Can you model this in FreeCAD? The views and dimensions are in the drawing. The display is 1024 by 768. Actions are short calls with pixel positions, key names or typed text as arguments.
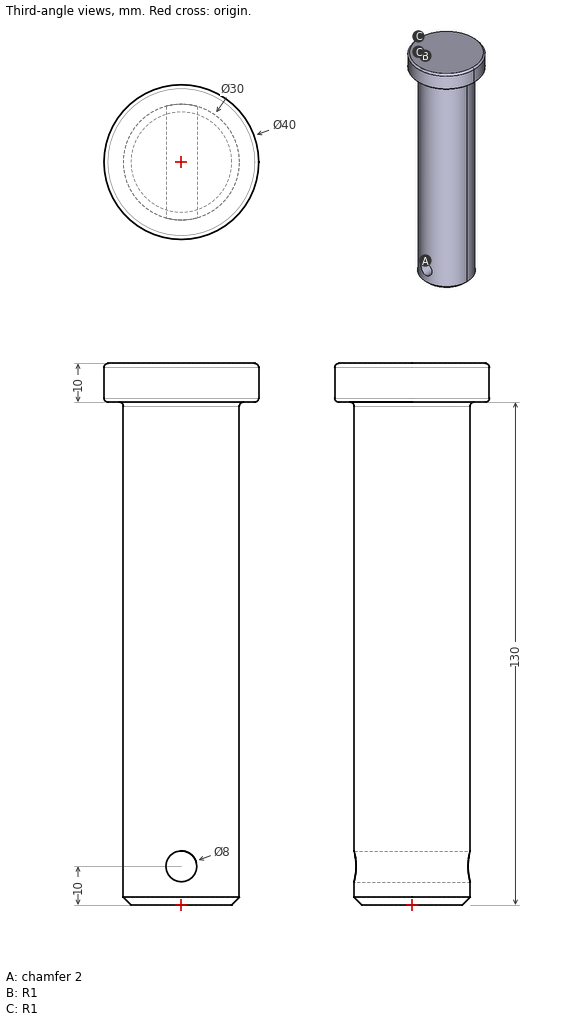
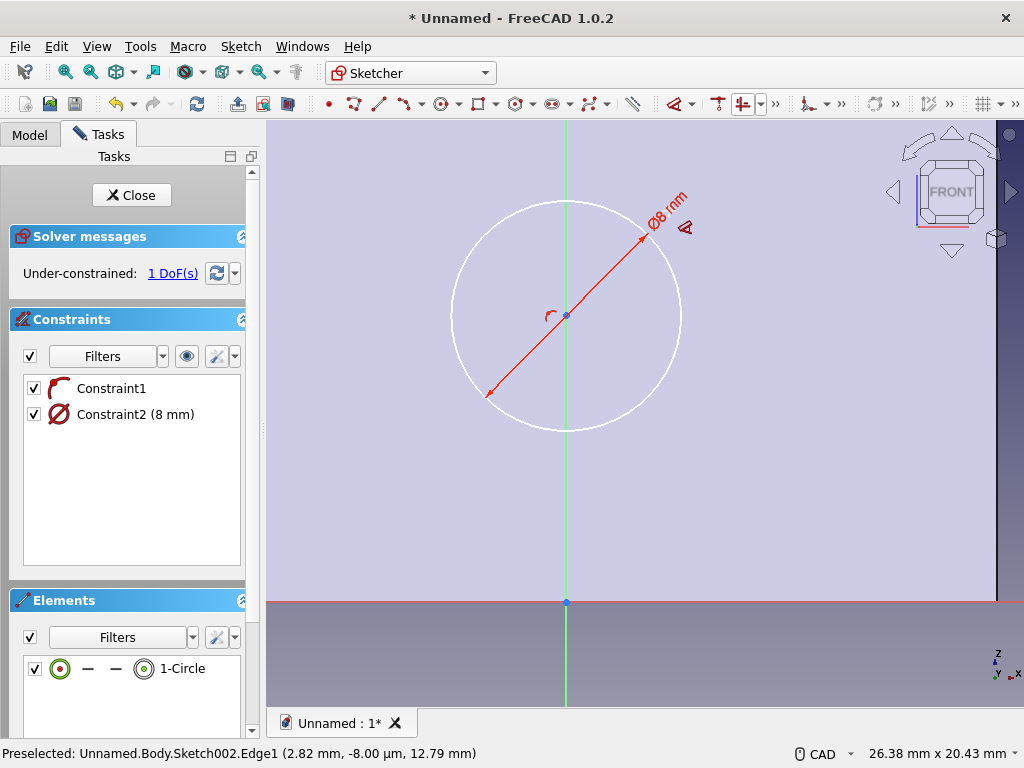
click(566, 316)
click(600, 459)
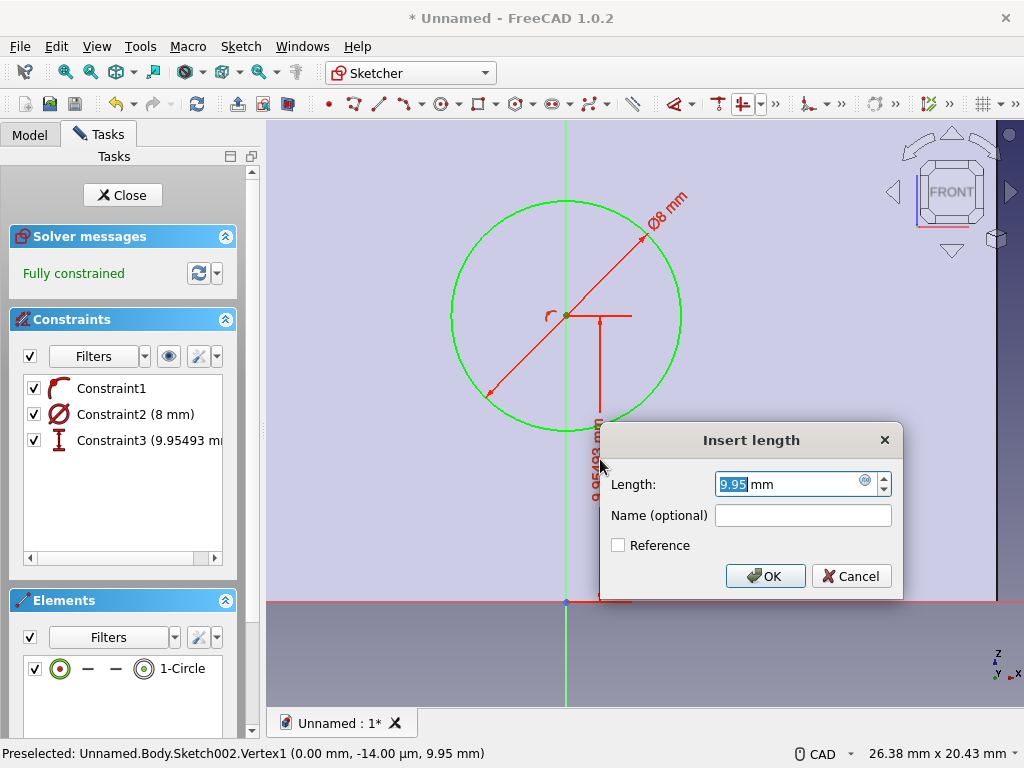
text(10)
key(Return)
key(Escape)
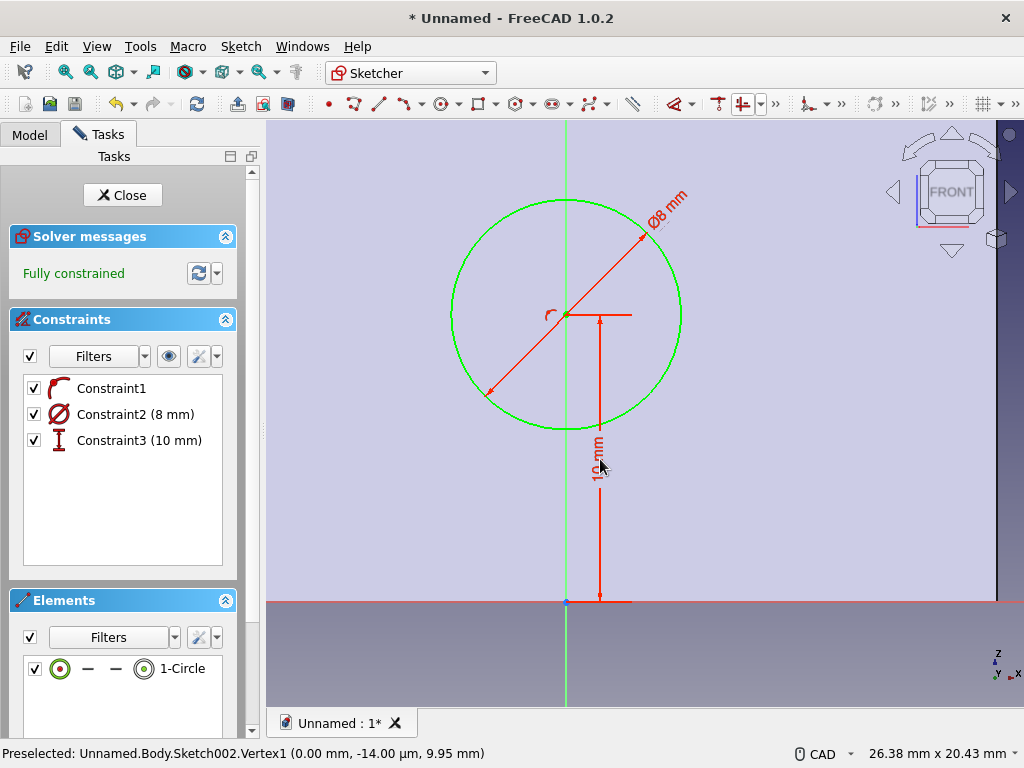
click(123, 195)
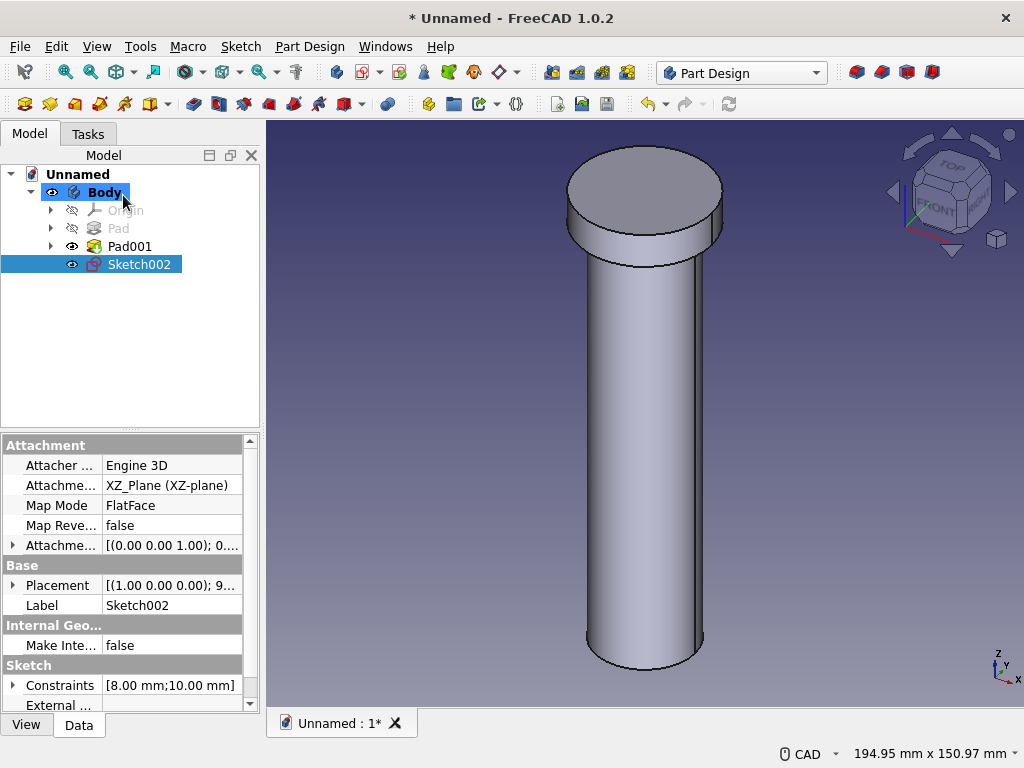
click(194, 104)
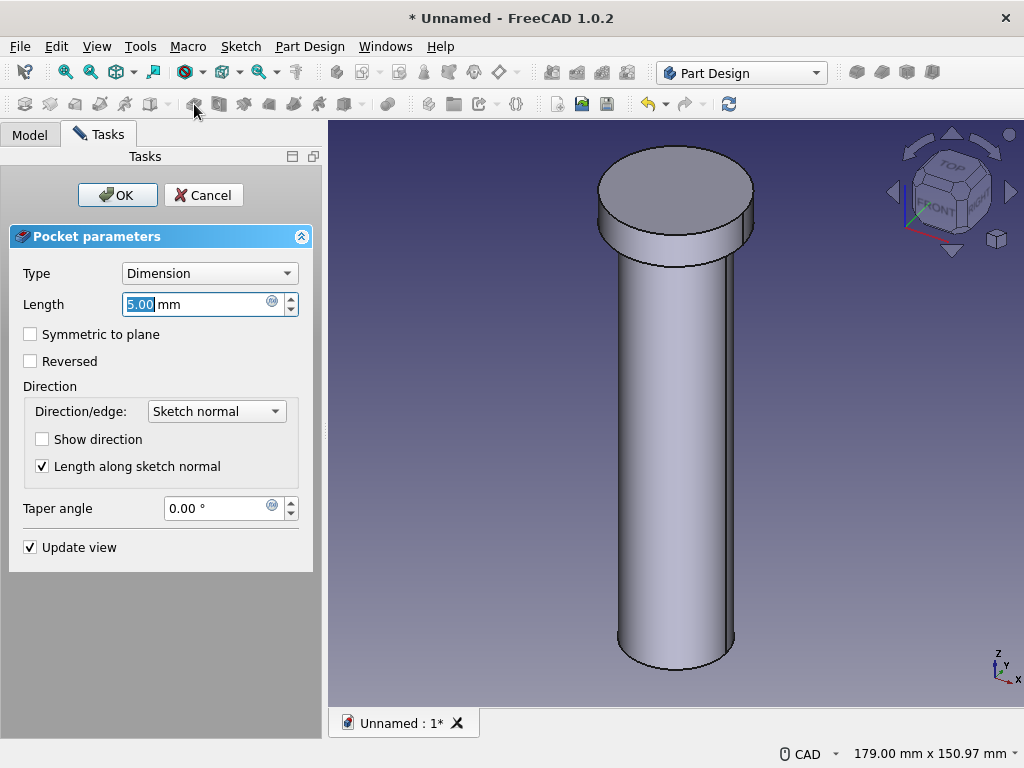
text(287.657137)
key(Tab)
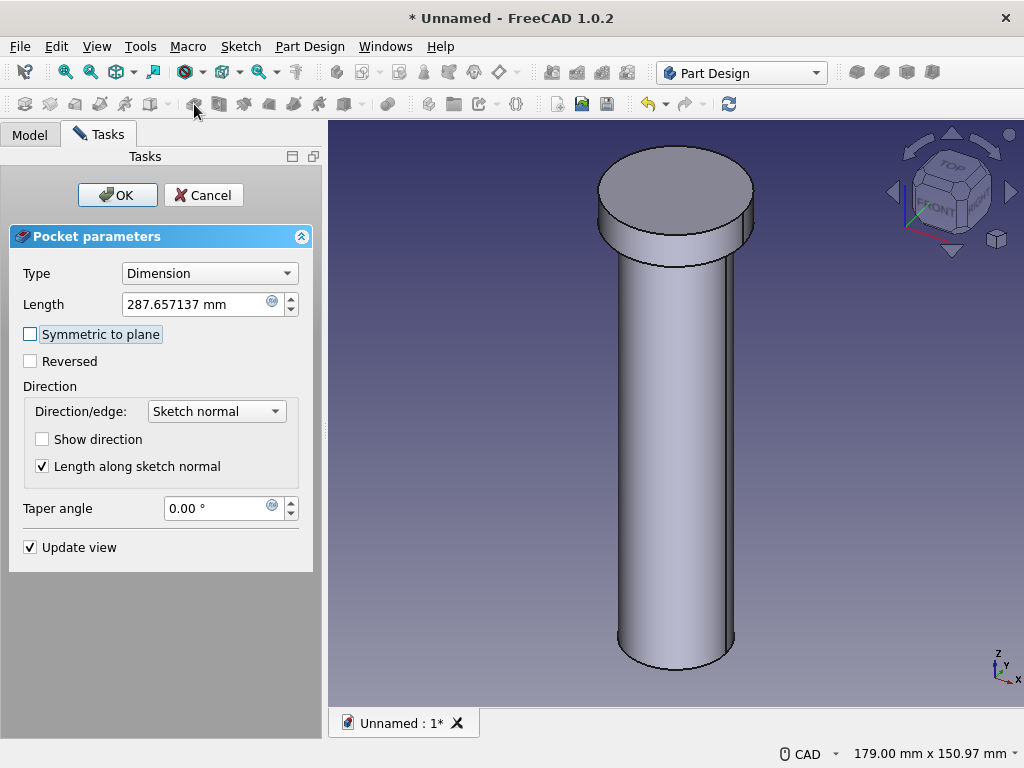
click(31, 334)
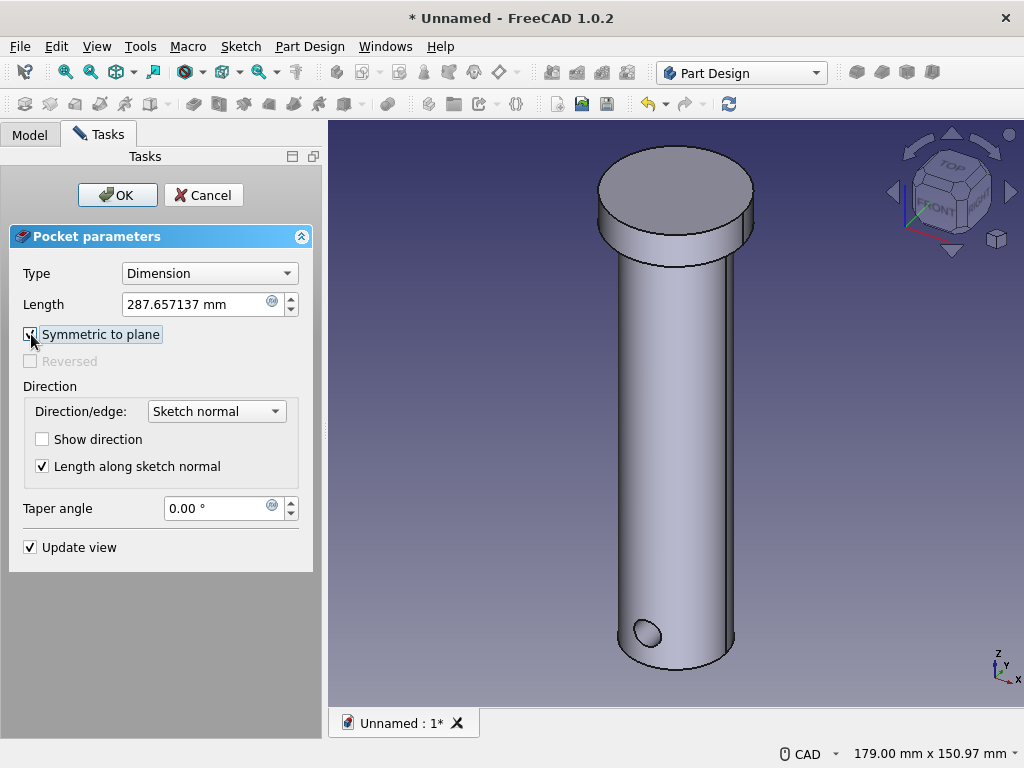
click(118, 195)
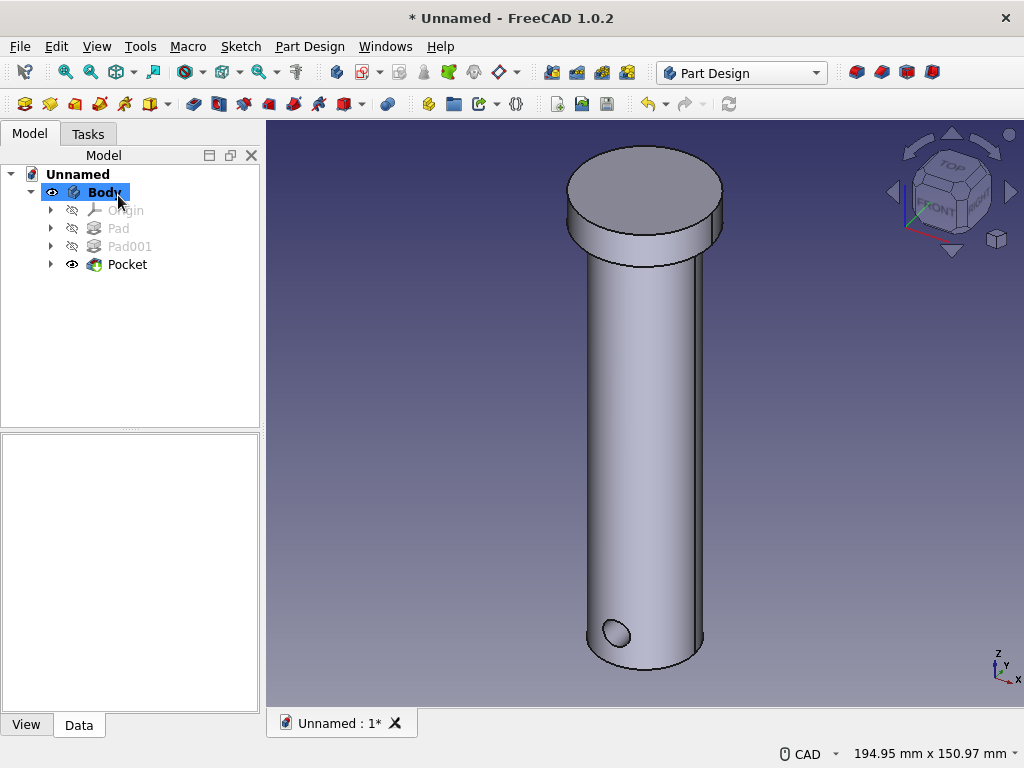
key(0)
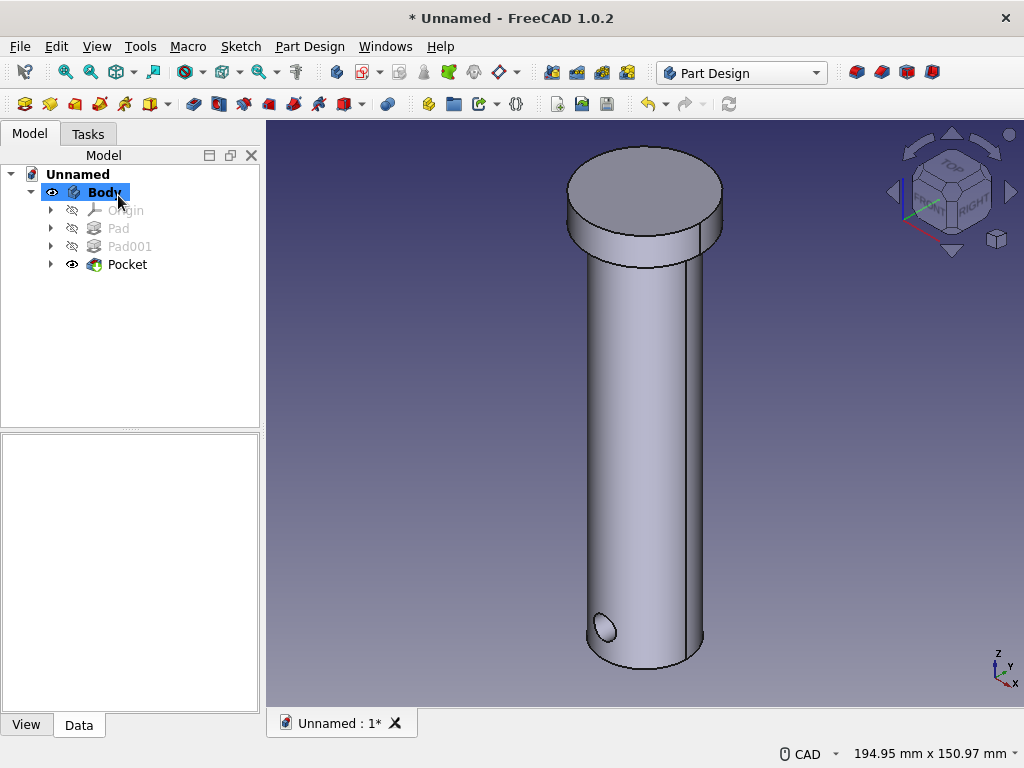
key(2)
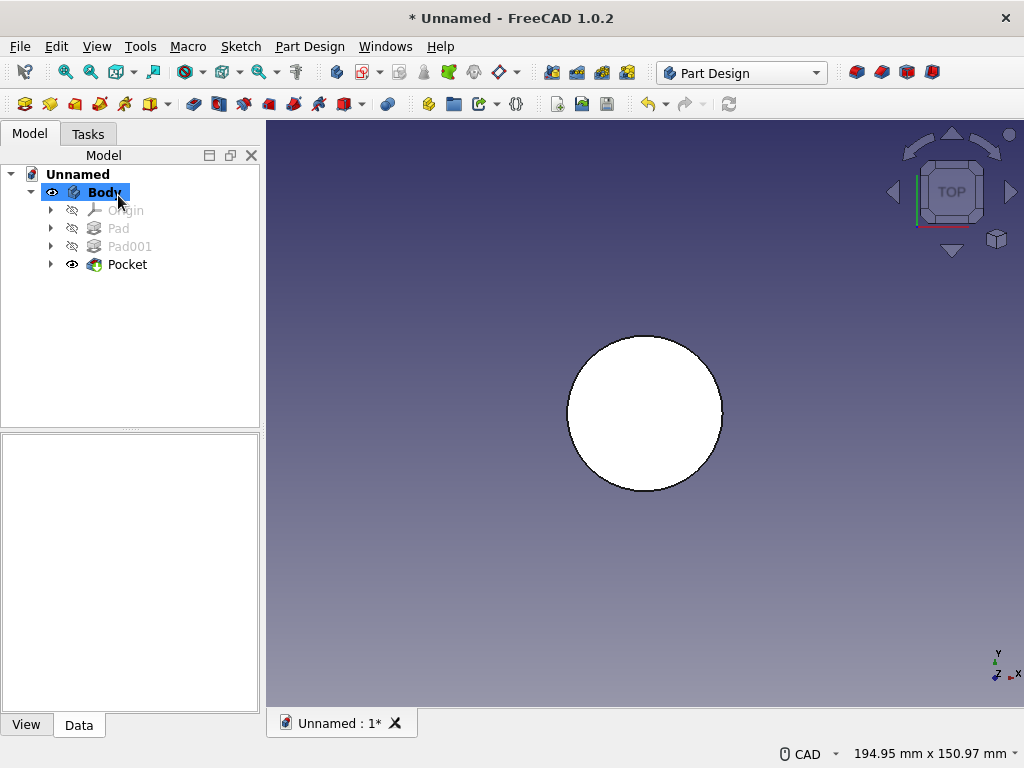
click(66, 72)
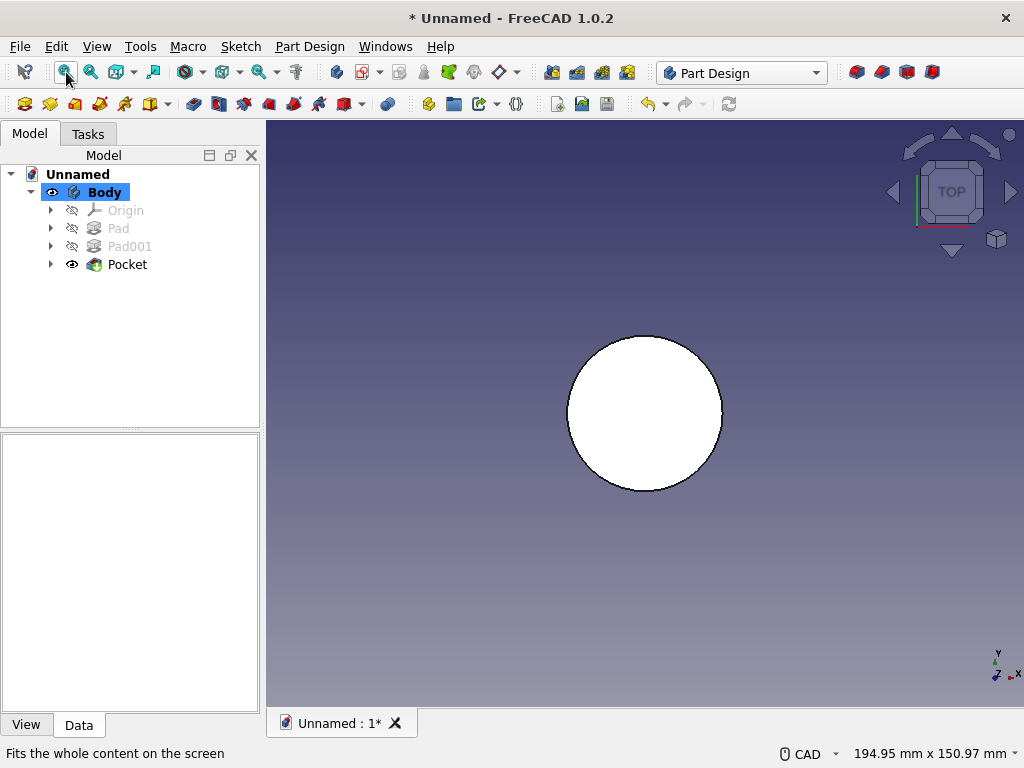
key(1)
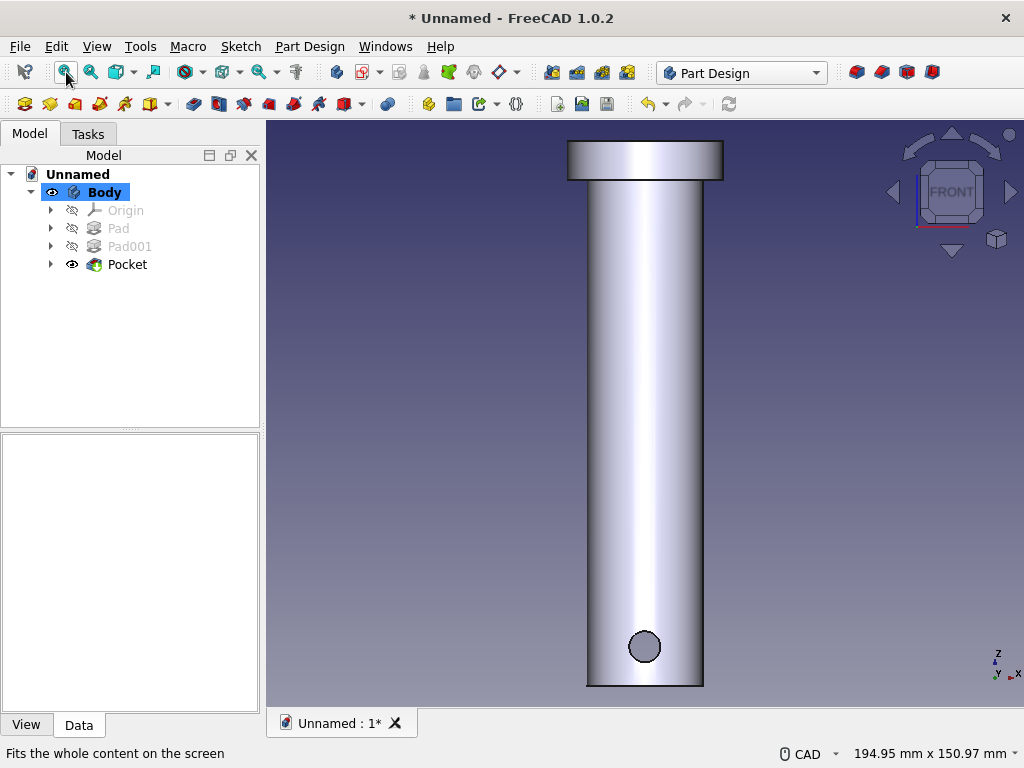
key(3)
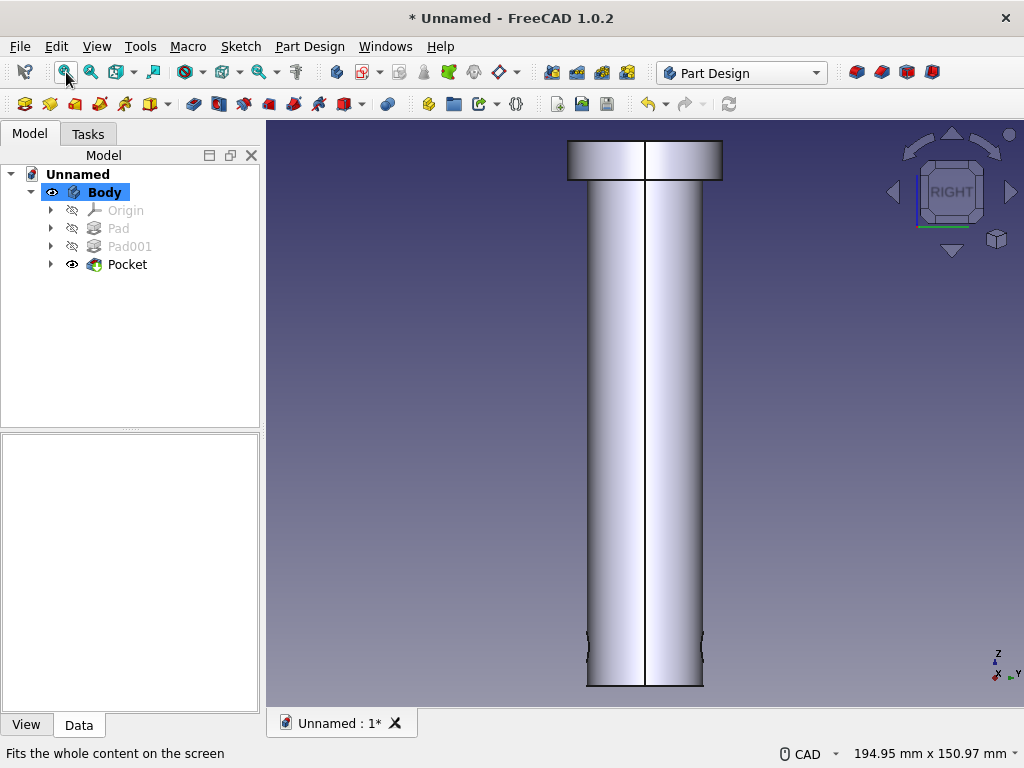
key(5)